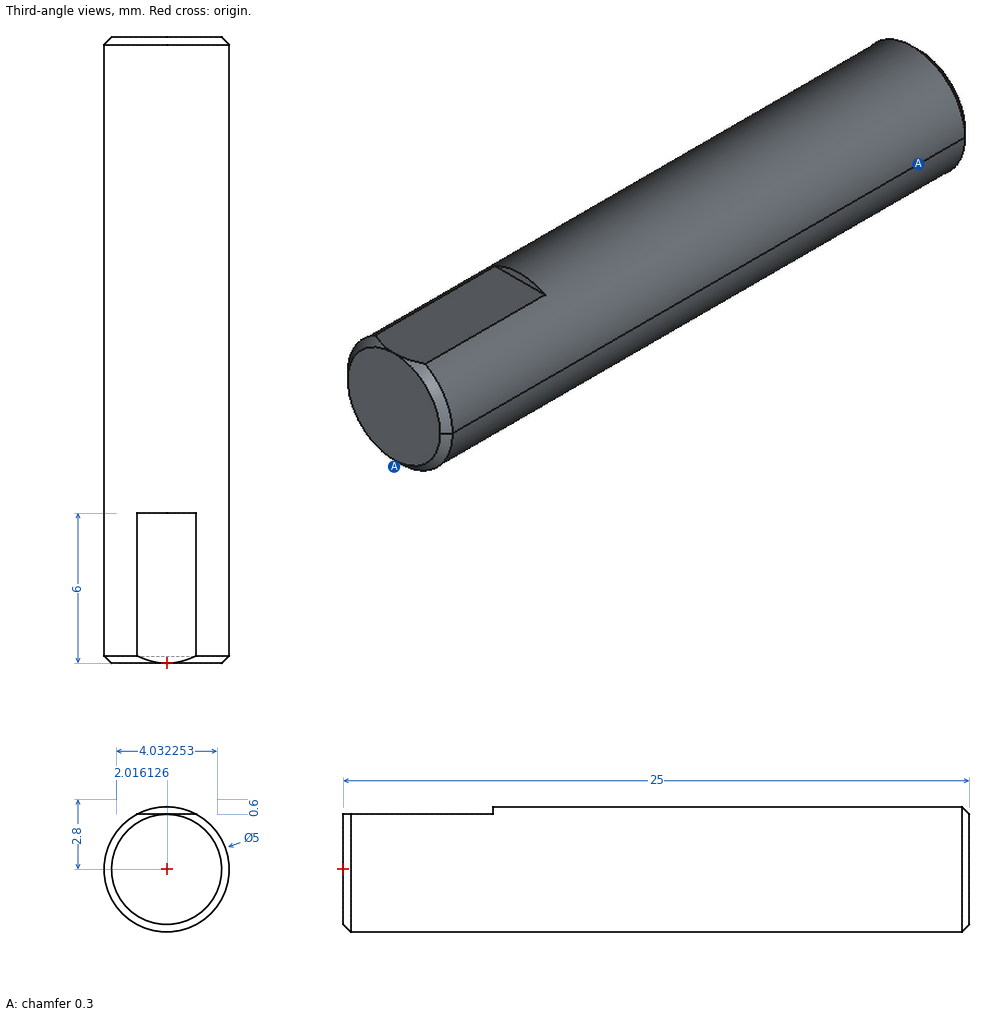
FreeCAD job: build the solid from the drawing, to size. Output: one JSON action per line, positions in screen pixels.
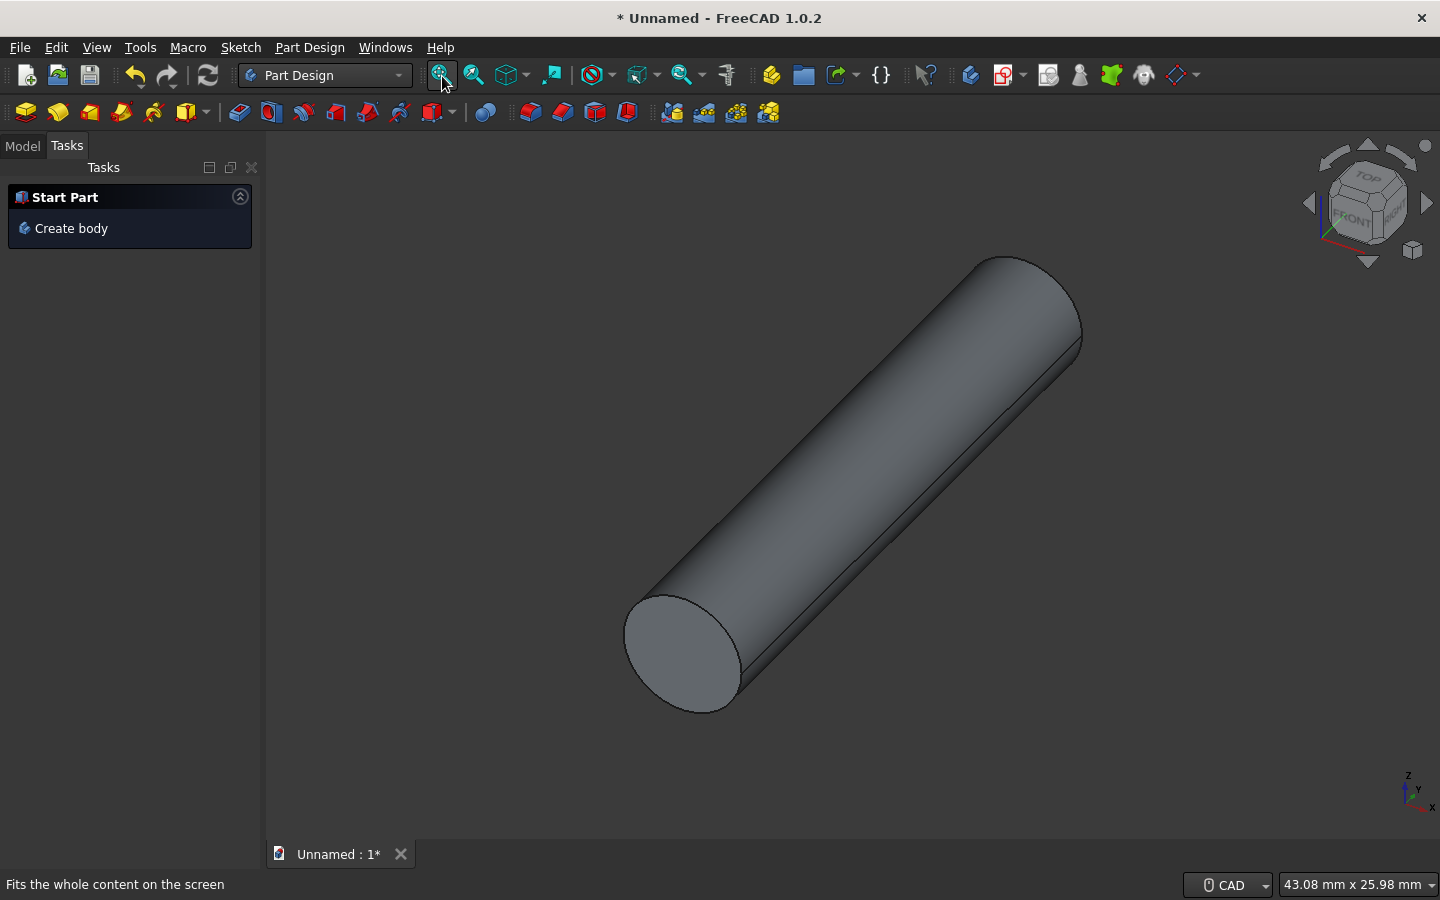
{"action": "left_click", "coordinate": [635, 605]}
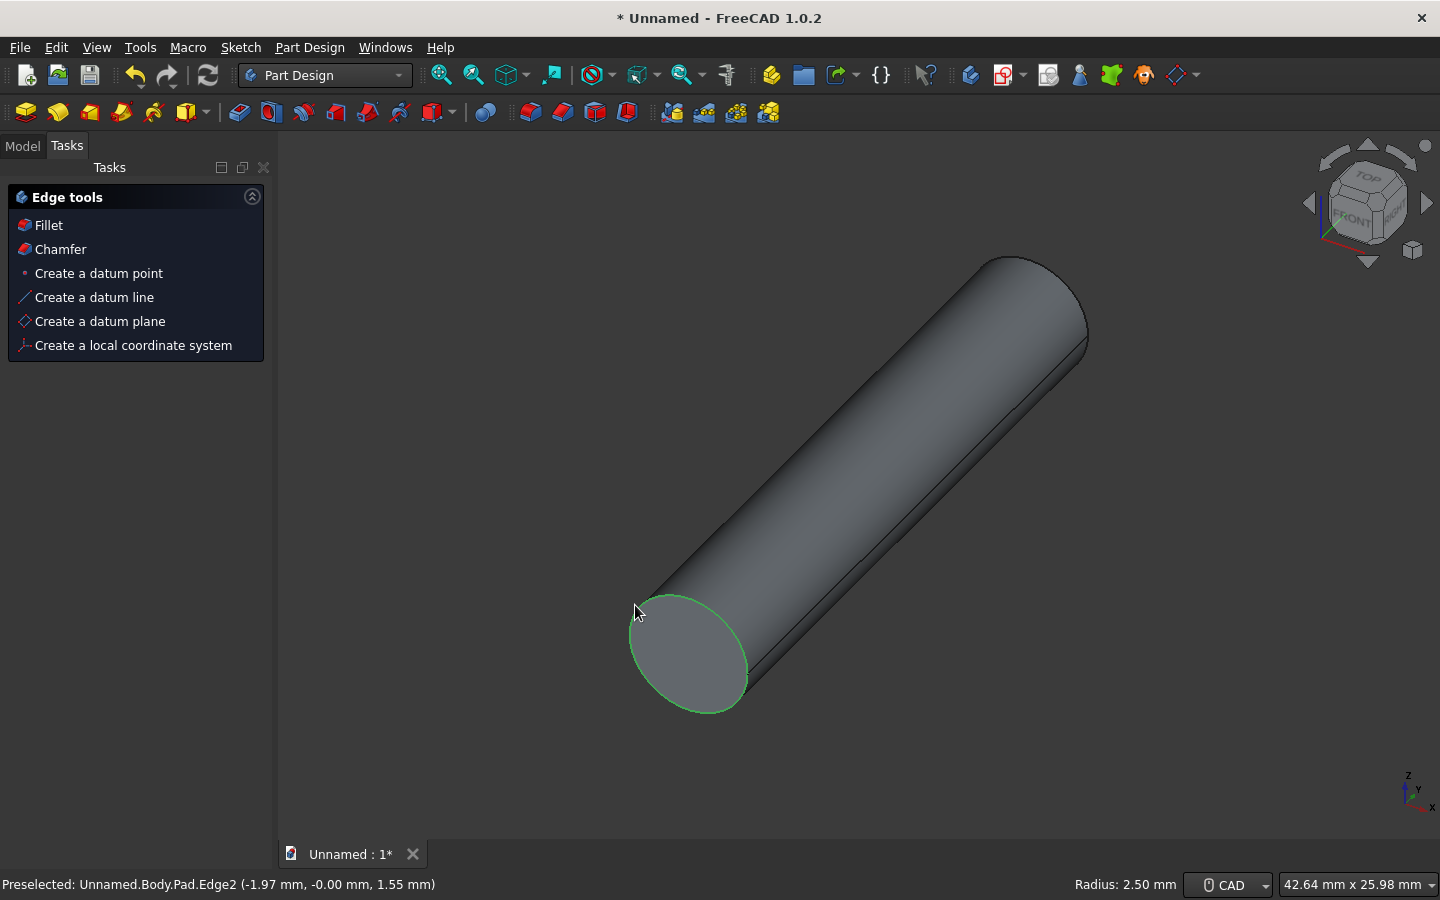
{"action": "key", "text": "0"}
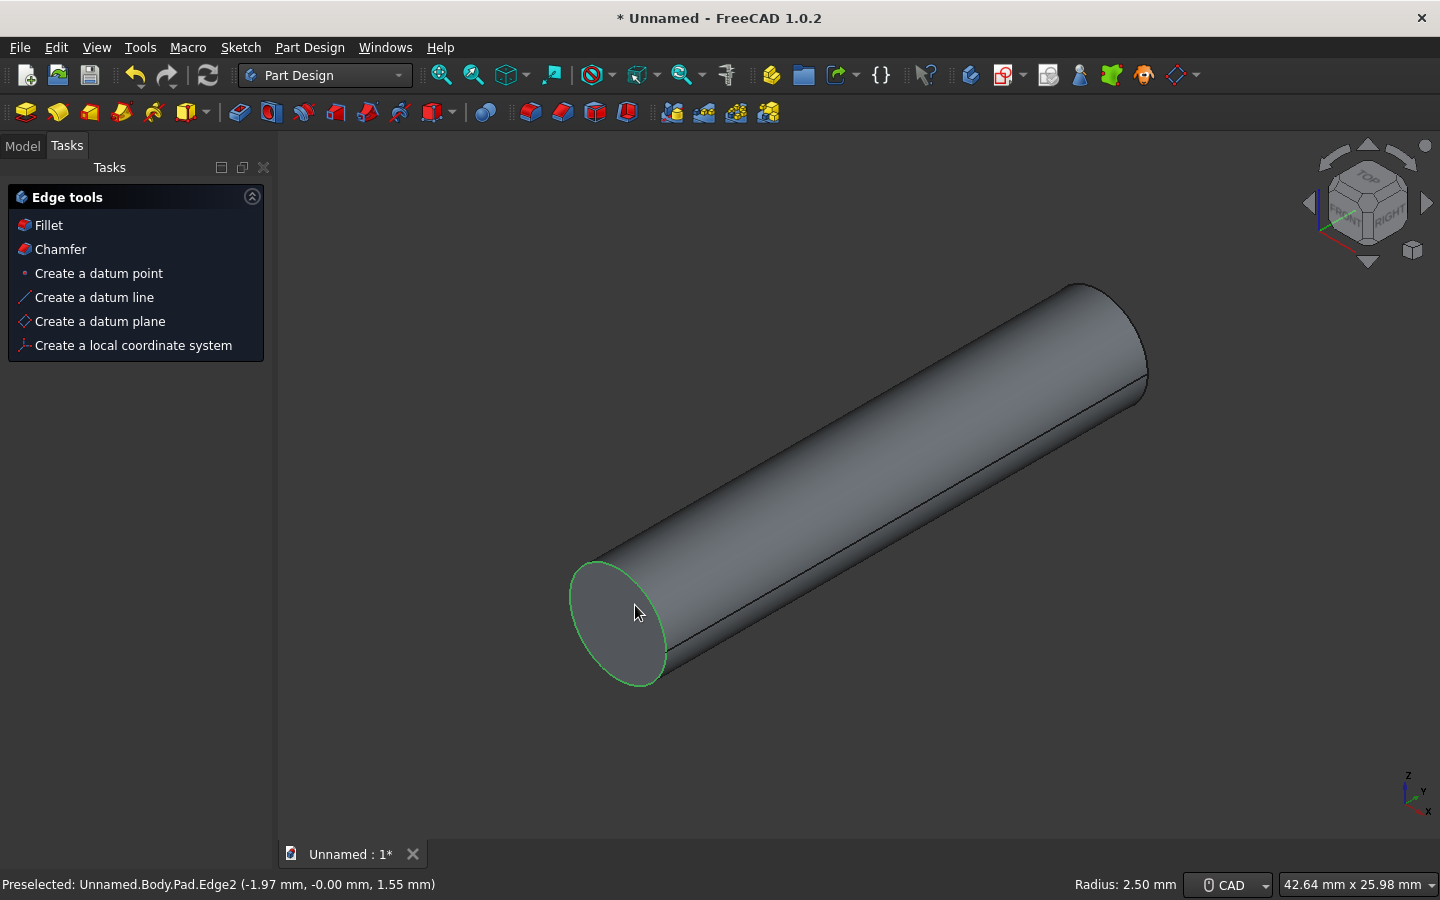
{"action": "key", "text": "2"}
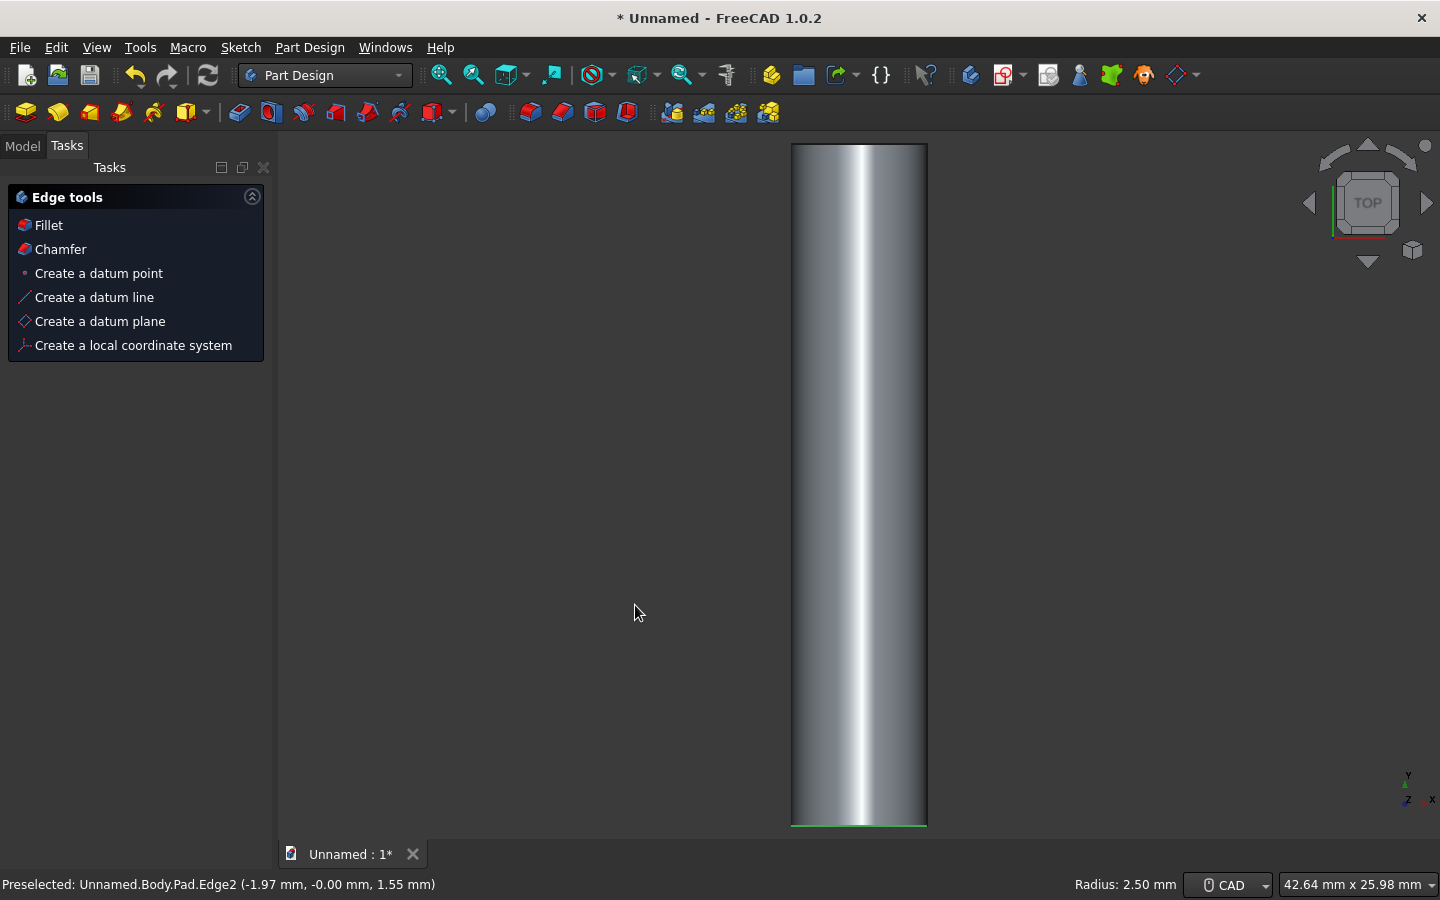
{"action": "key", "text": "1"}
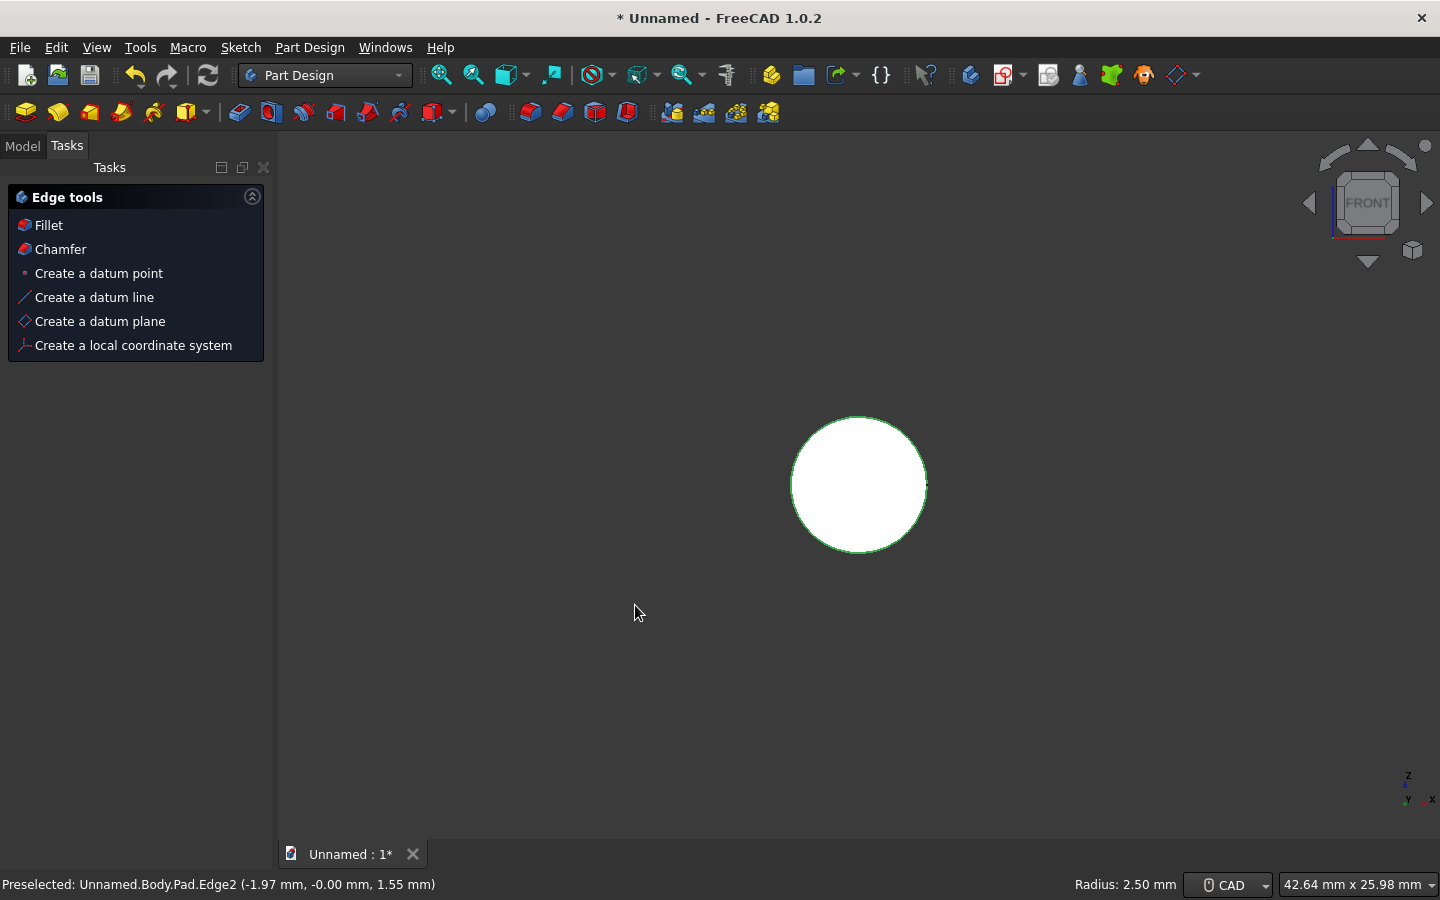
{"action": "left_click", "coordinate": [442, 76]}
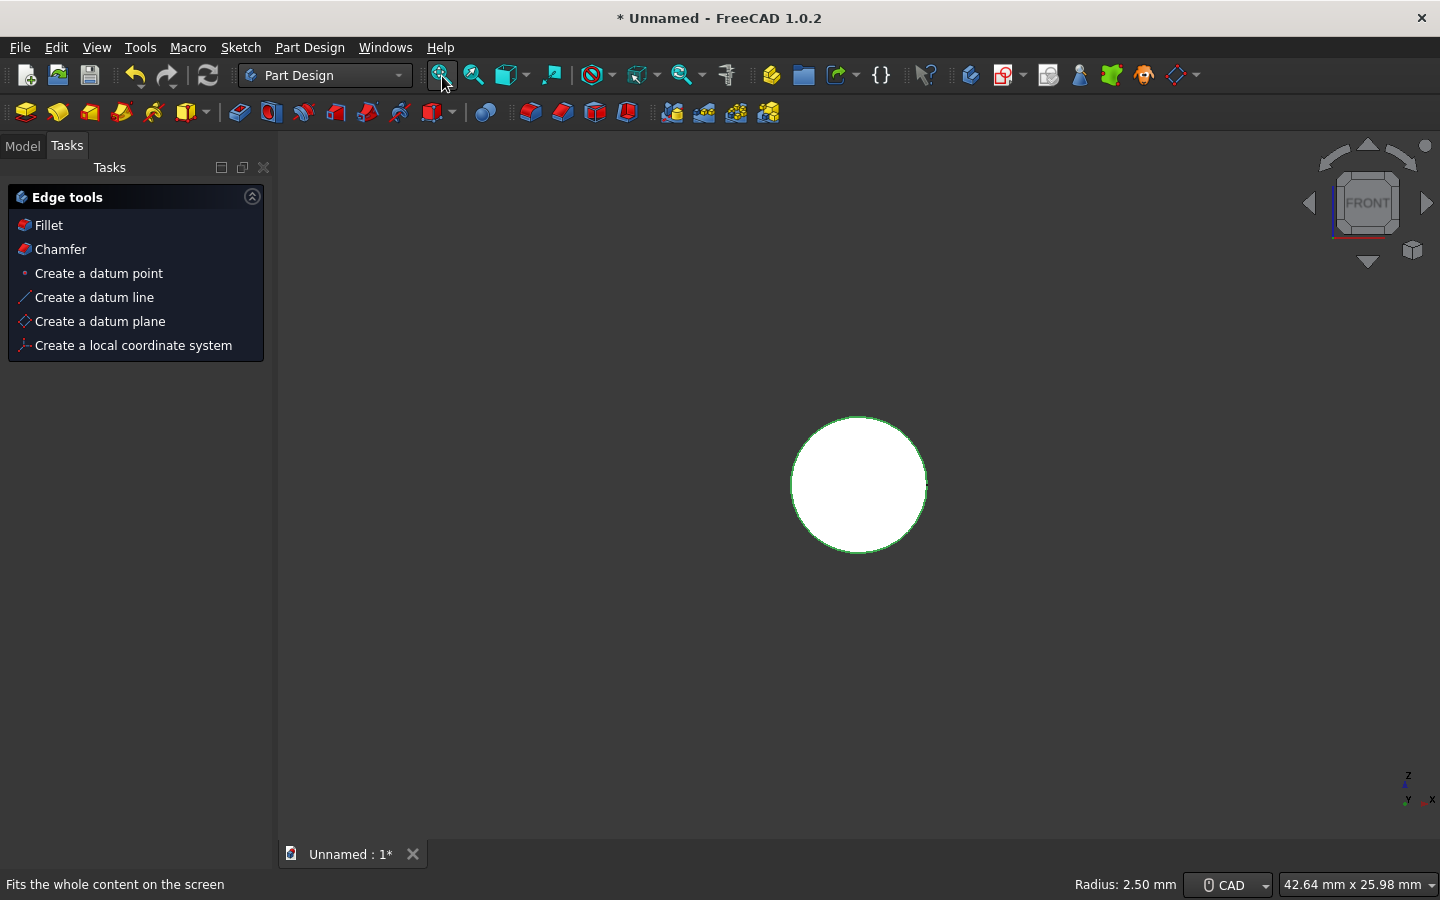
{"action": "key", "text": "3"}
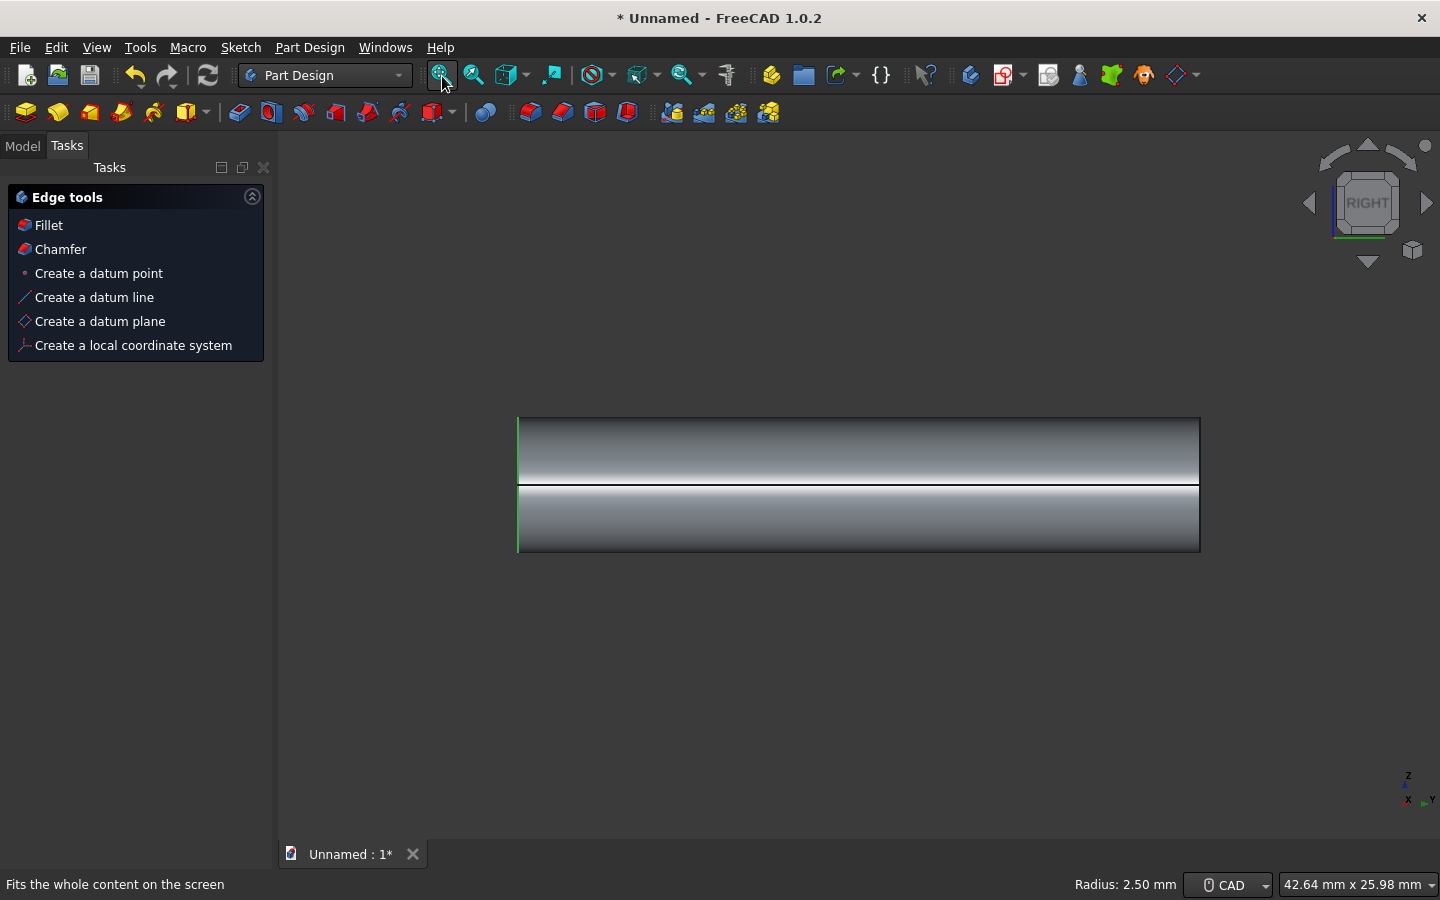
{"action": "left_click", "coordinate": [1200, 444], "text": "ctrl"}